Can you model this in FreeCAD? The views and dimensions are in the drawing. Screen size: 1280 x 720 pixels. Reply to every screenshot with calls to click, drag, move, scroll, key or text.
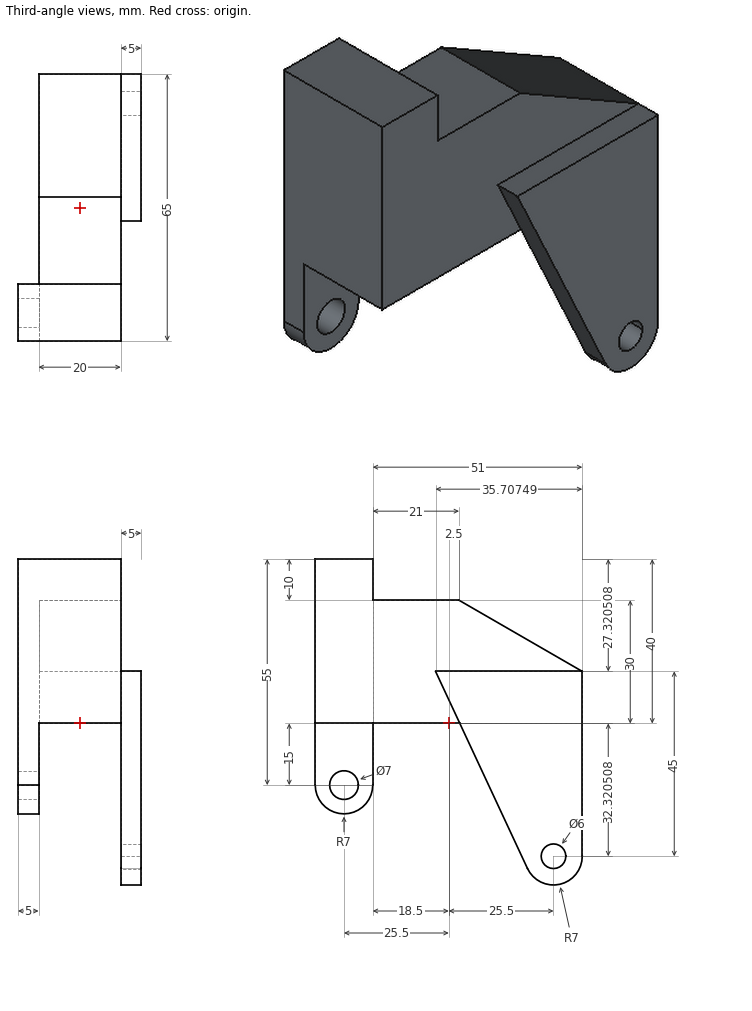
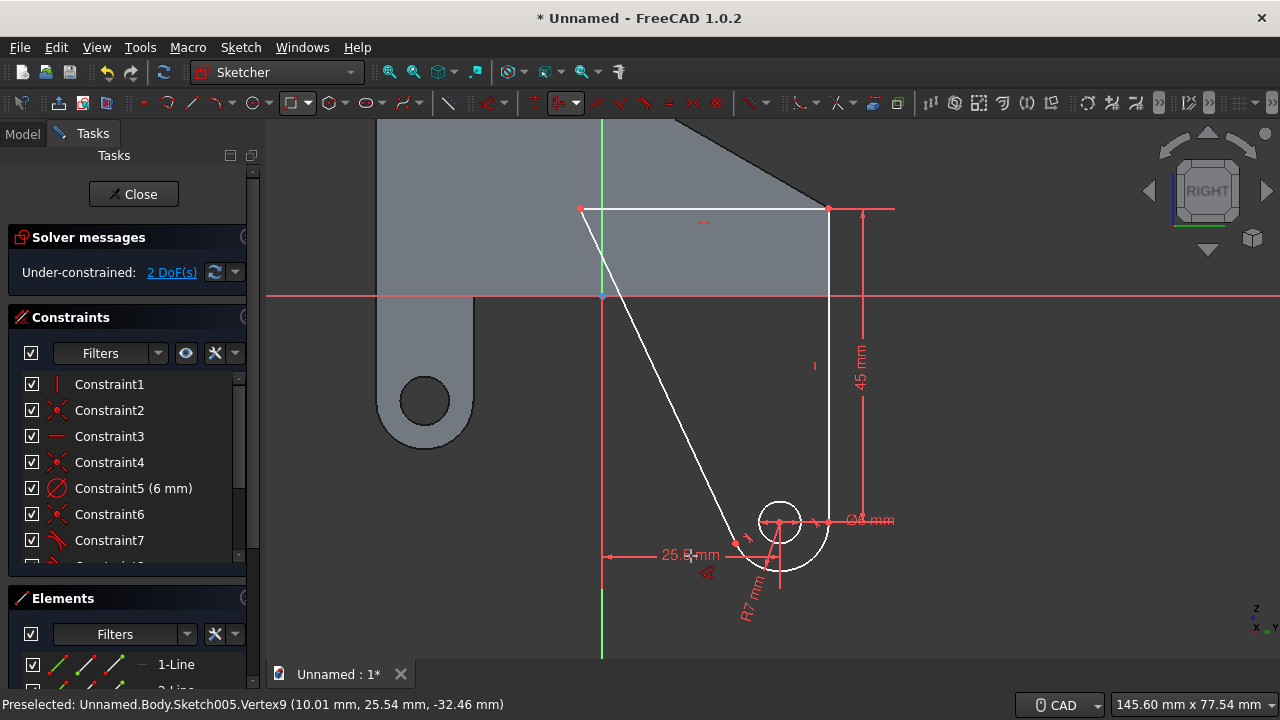
click(754, 209)
click(704, 175)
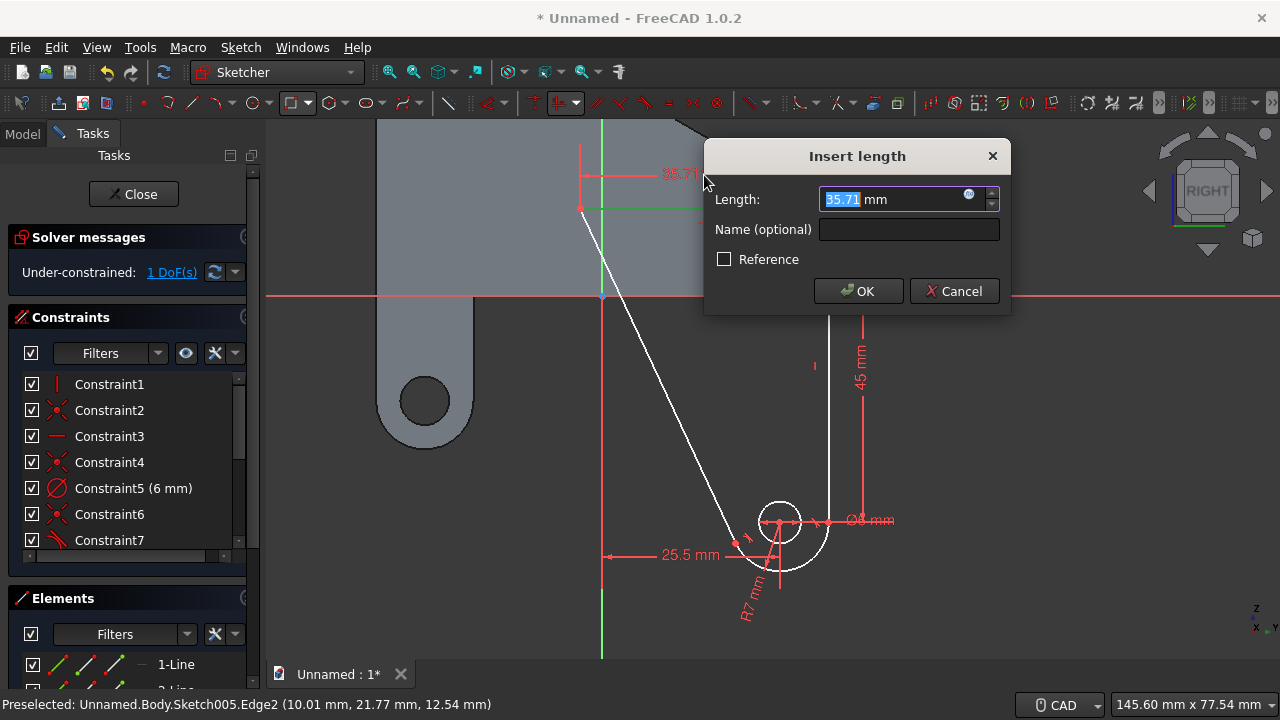
text(35.70749)
key(Return)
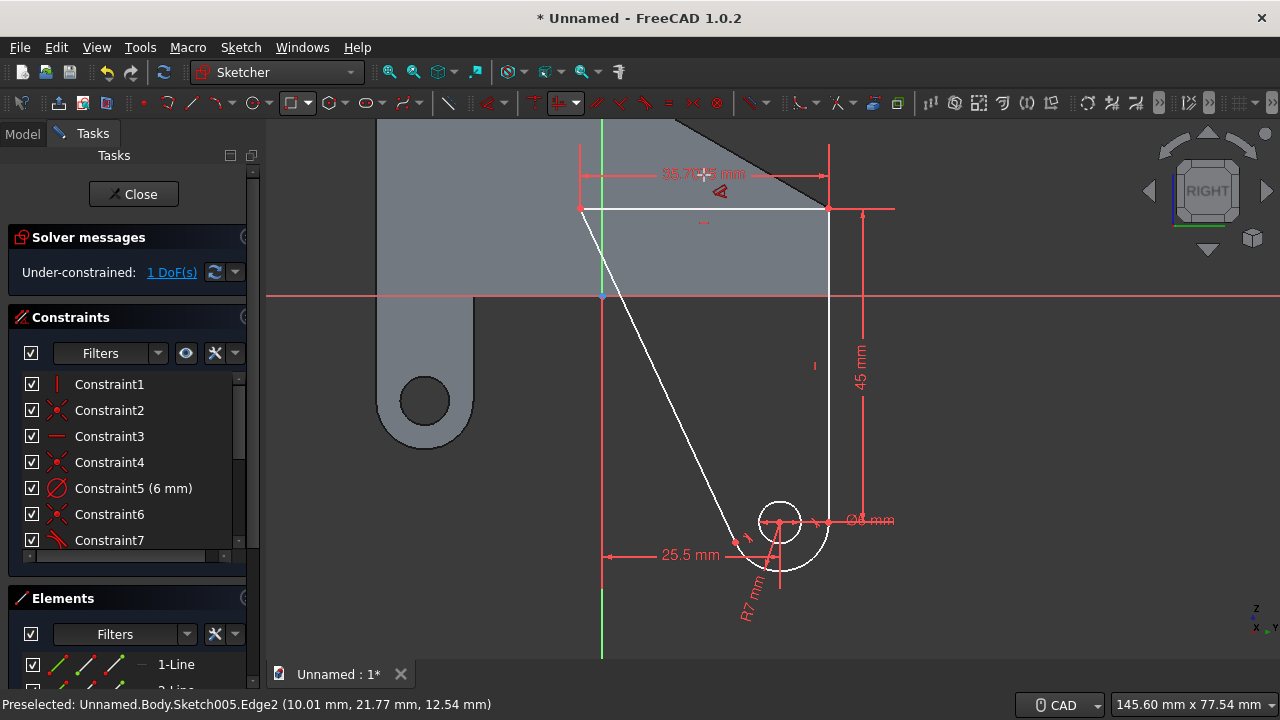
click(780, 522)
click(568, 409)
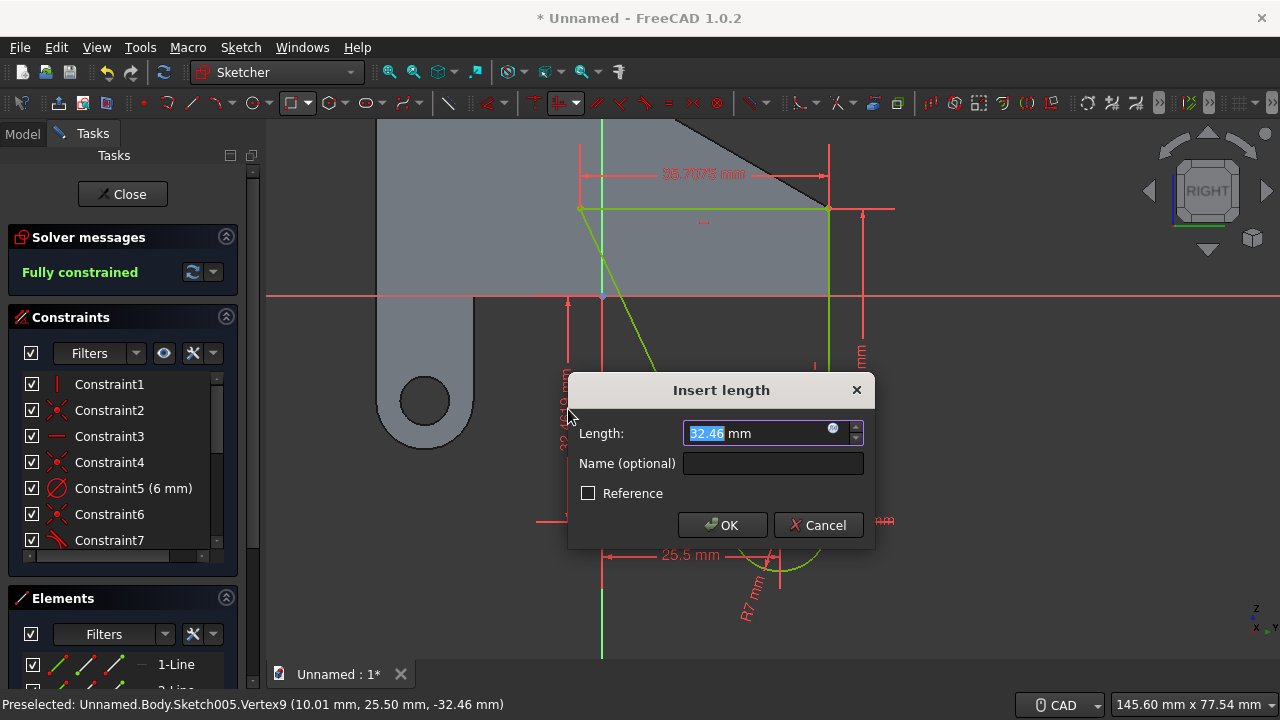
text(32.320508)
key(Return)
key(Escape)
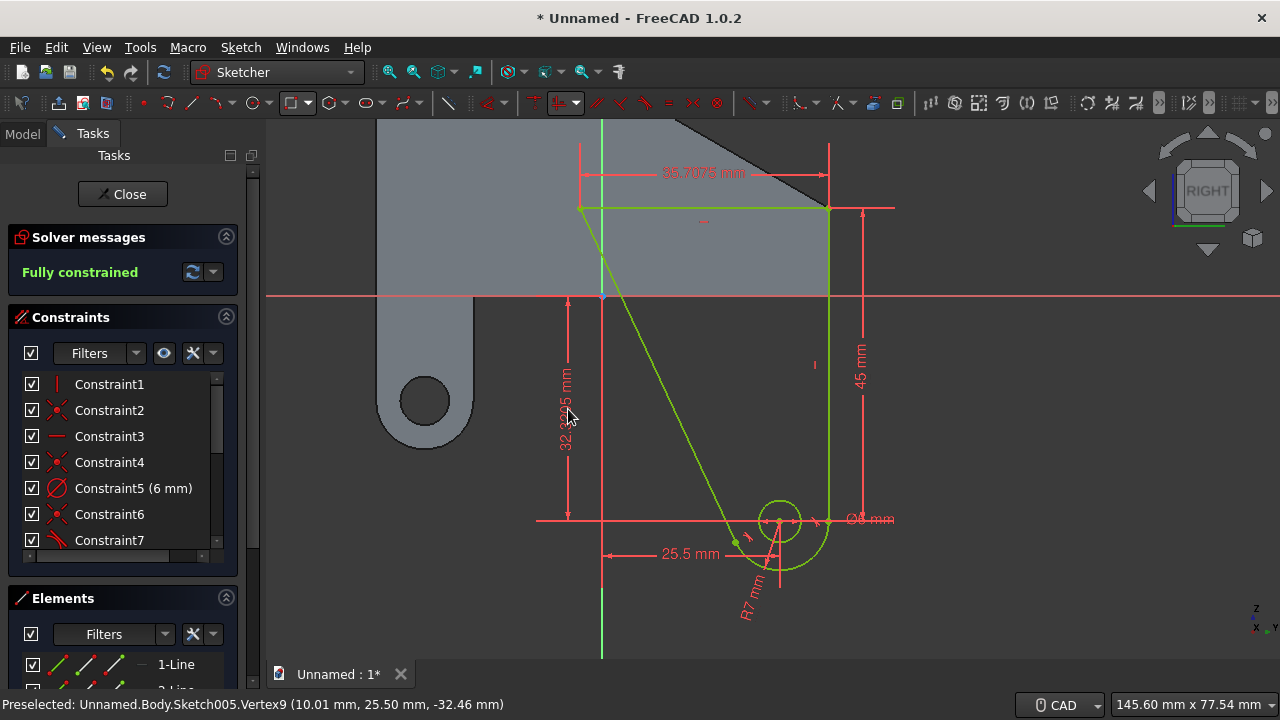
click(123, 194)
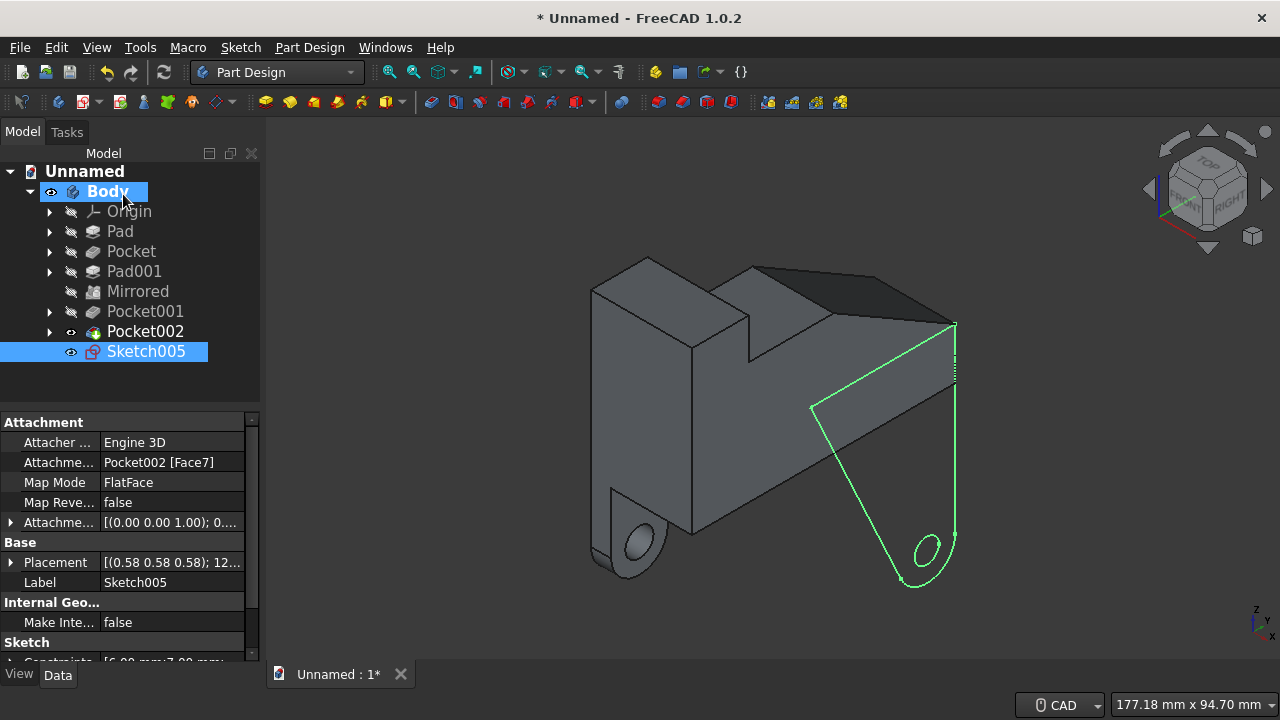
click(266, 102)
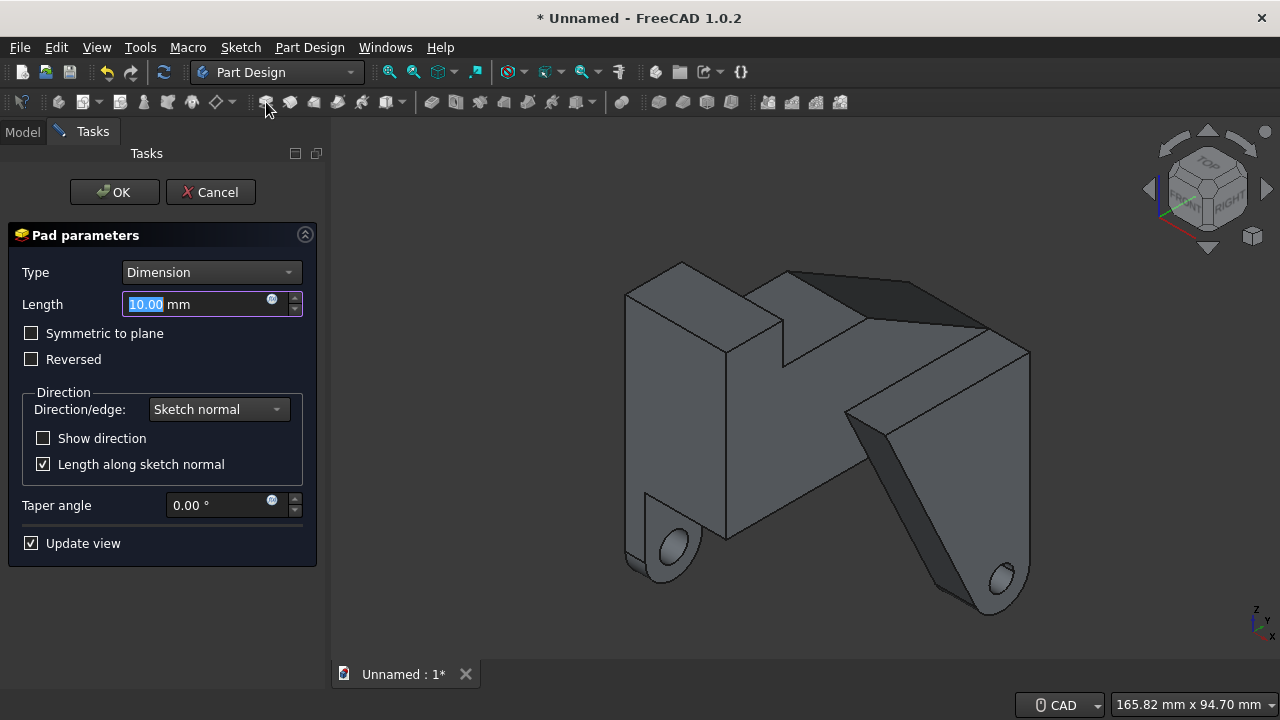
text(5)
key(Tab)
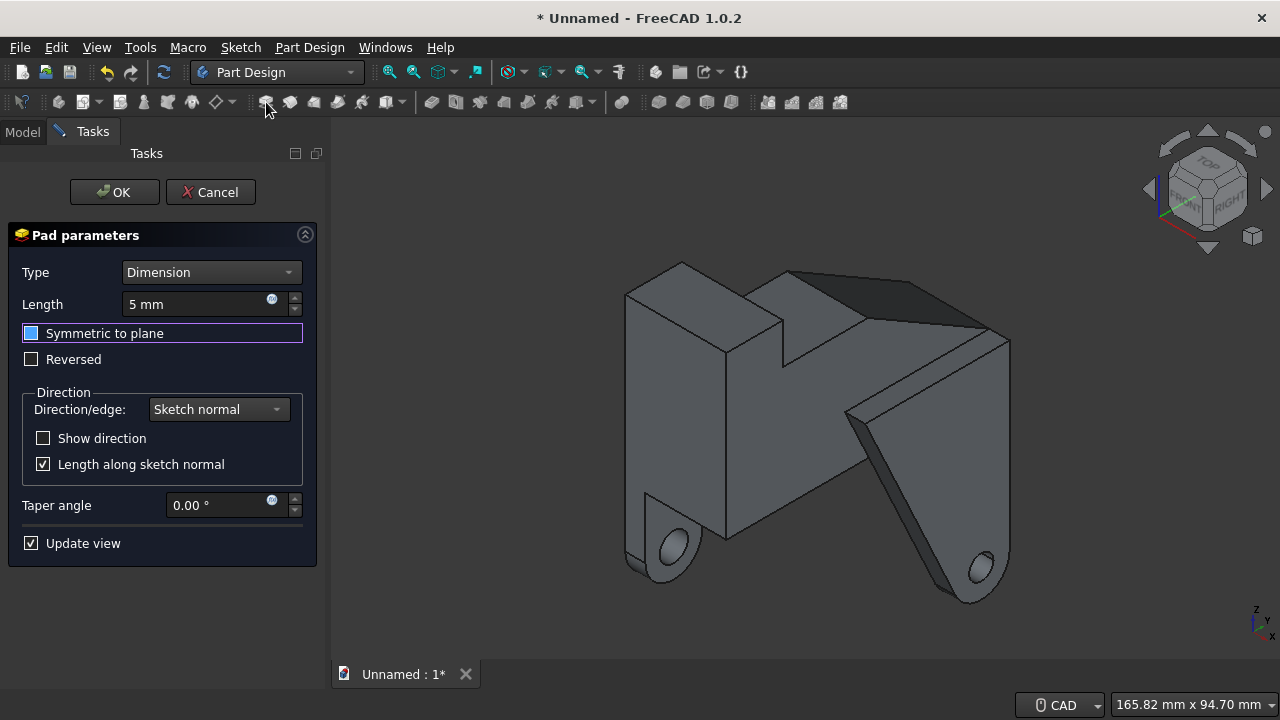
click(115, 192)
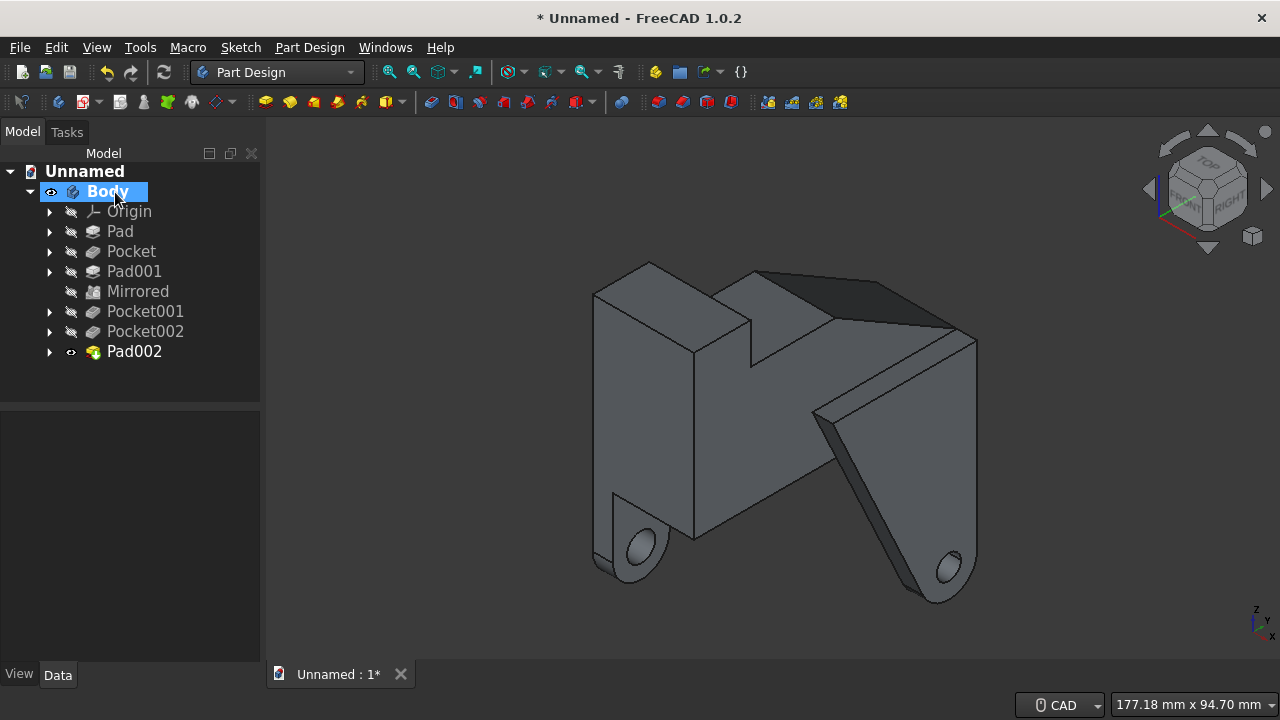
key(v)
key(f)